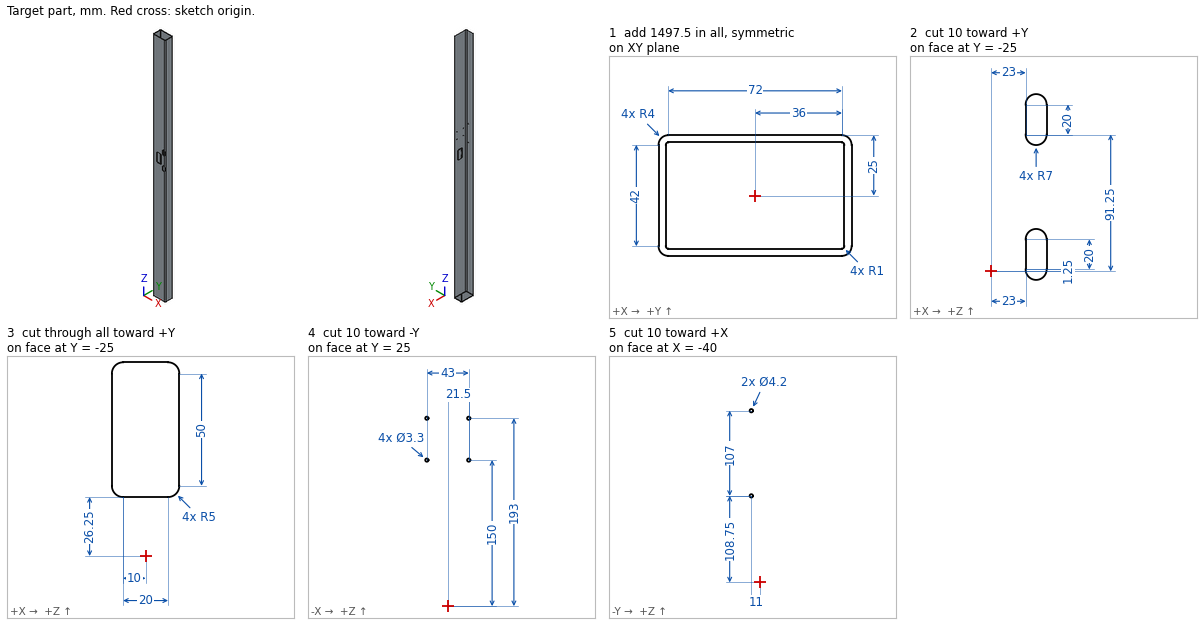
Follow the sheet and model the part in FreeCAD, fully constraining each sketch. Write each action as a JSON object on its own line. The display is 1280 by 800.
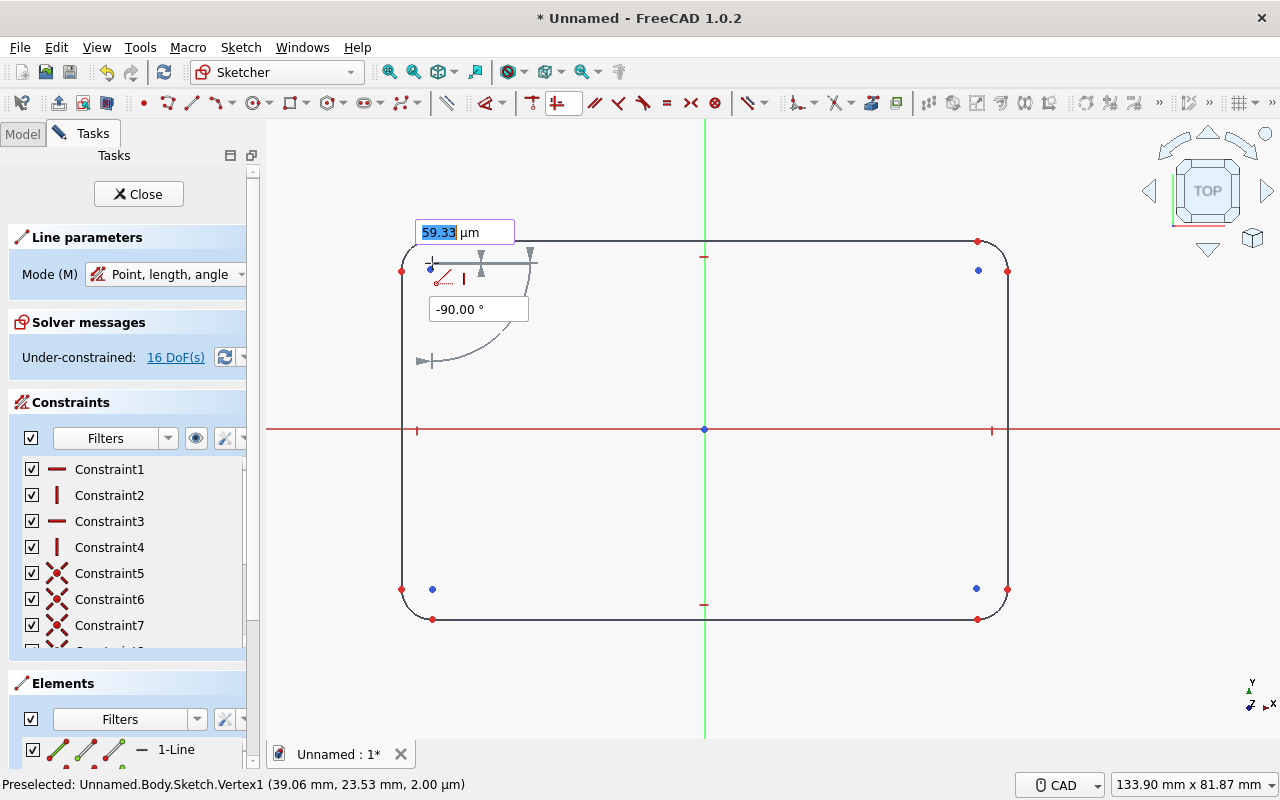
{"action": "scroll", "coordinate": [977, 263], "scroll_direction": "up", "scroll_amount": 4}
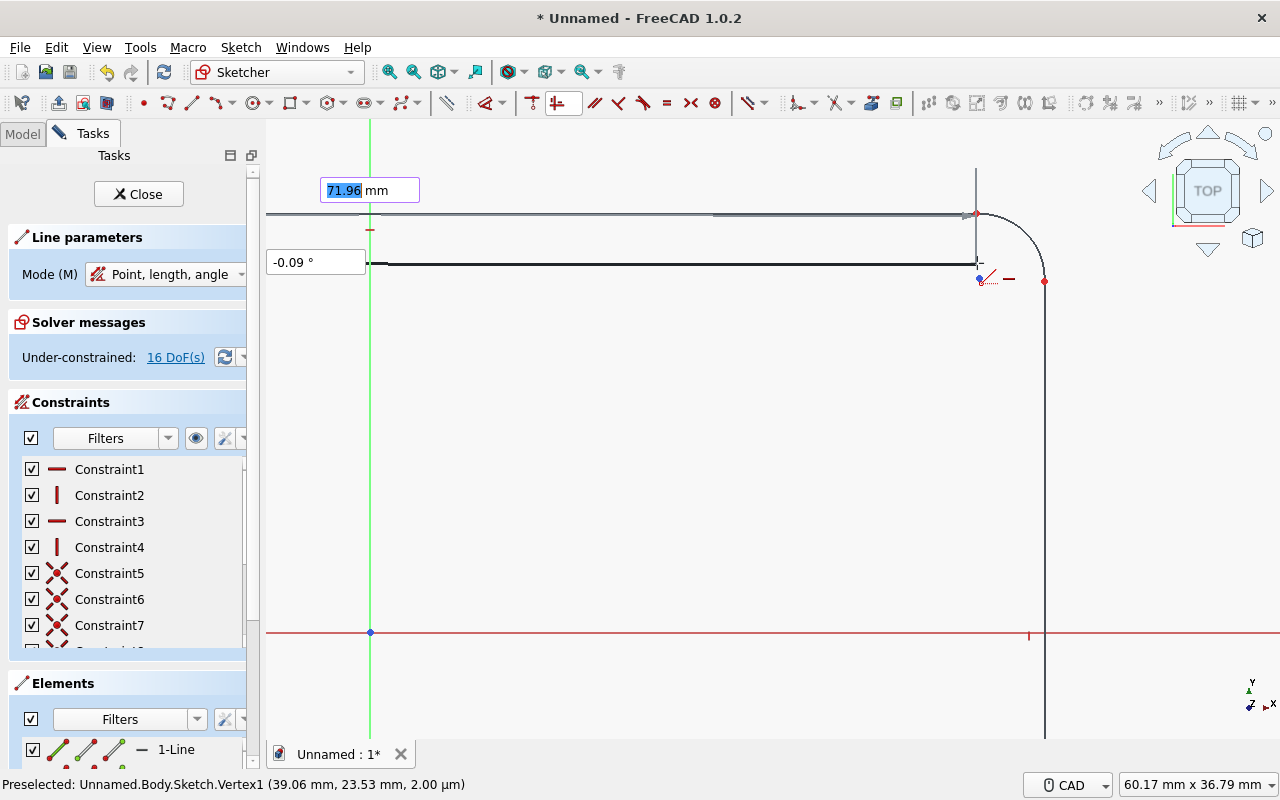
{"action": "left_click", "coordinate": [977, 262]}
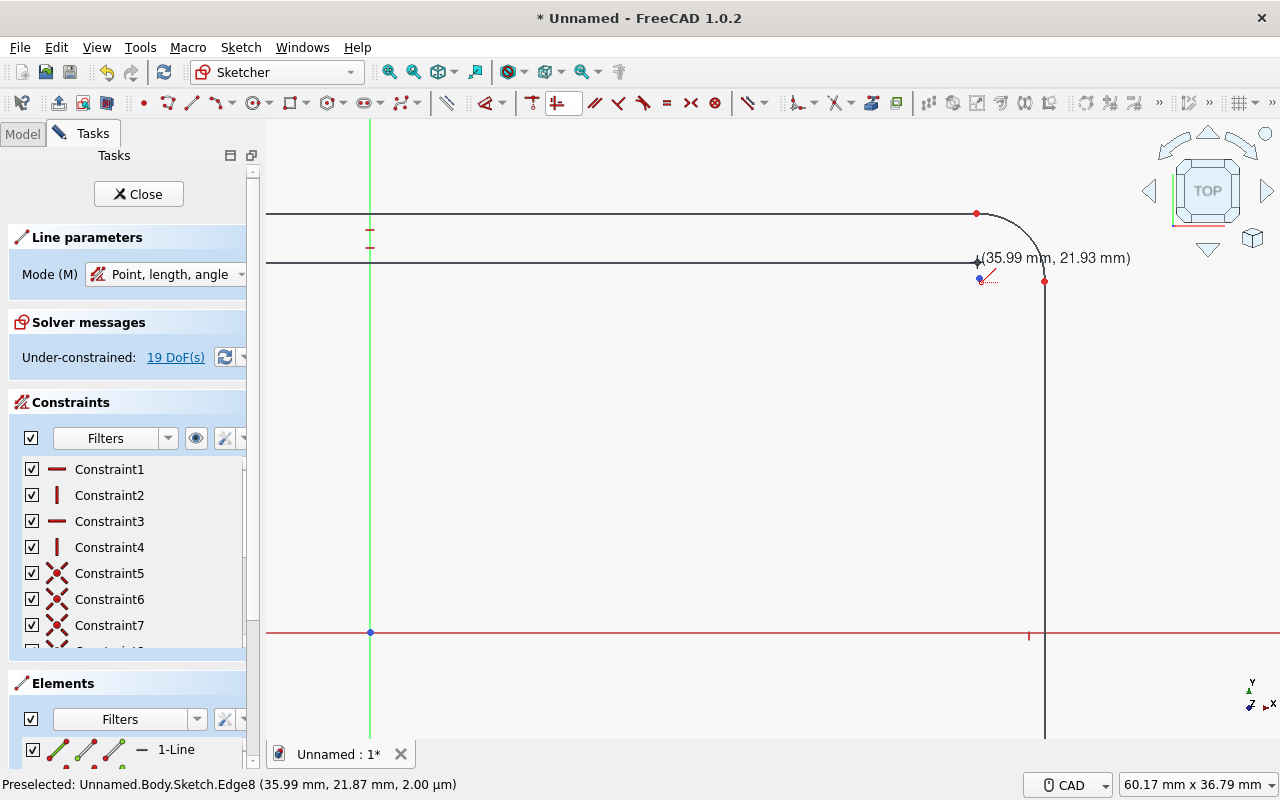
{"action": "left_click", "coordinate": [994, 279]}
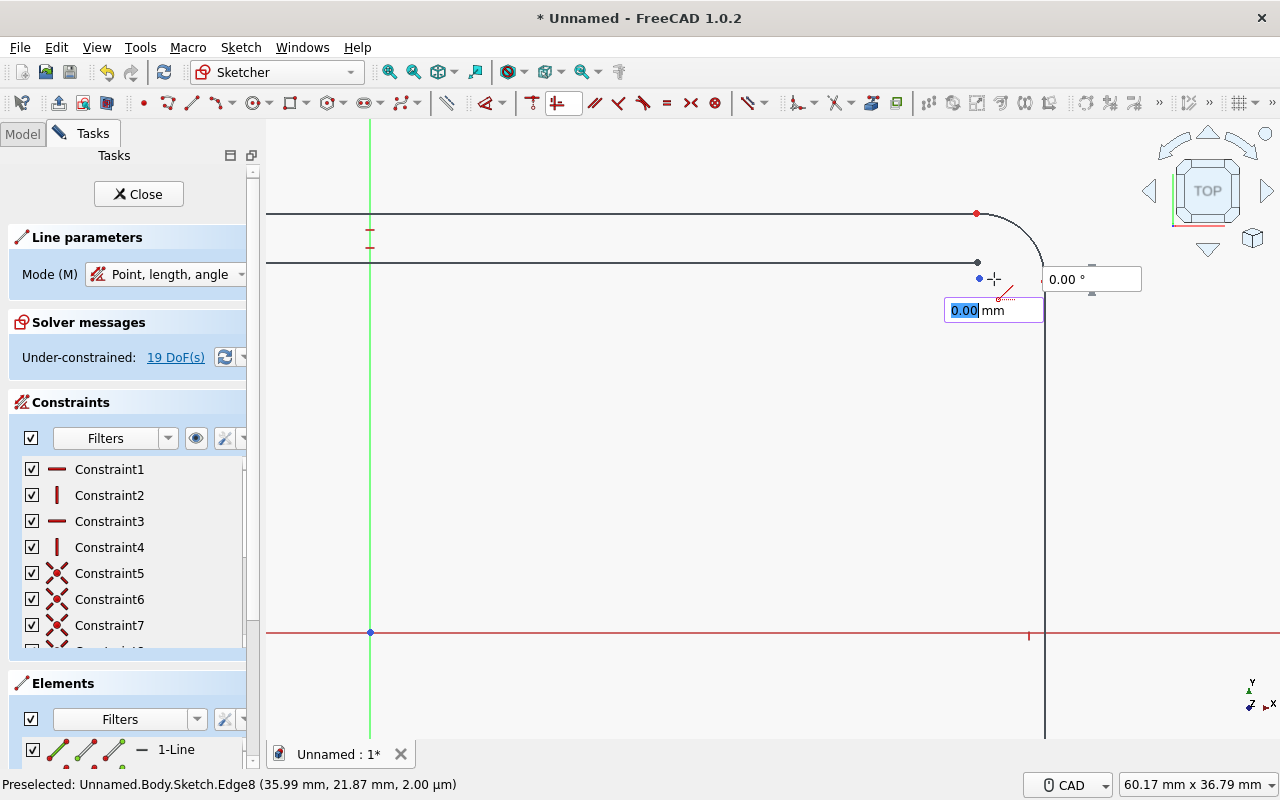
{"action": "scroll", "coordinate": [977, 263], "scroll_direction": "down", "scroll_amount": 4}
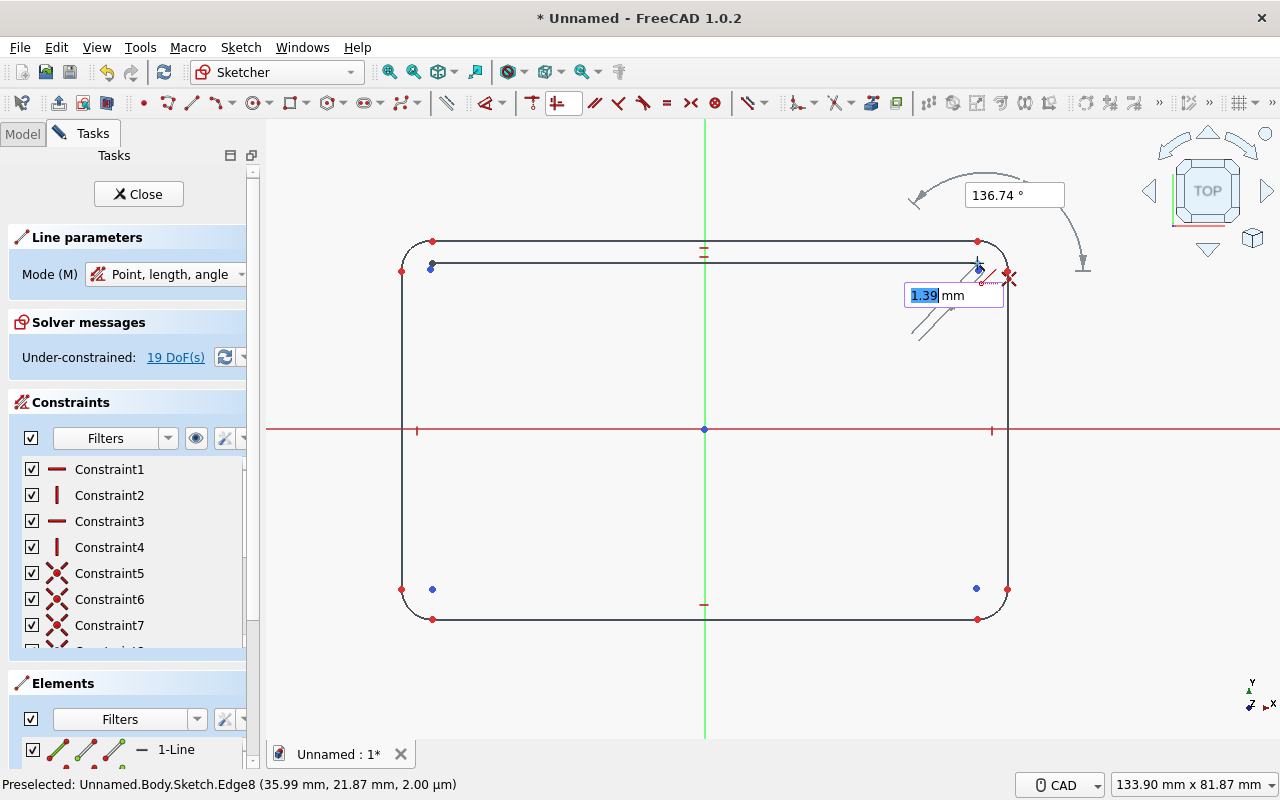
{"action": "scroll", "coordinate": [985, 588], "scroll_direction": "up", "scroll_amount": 4}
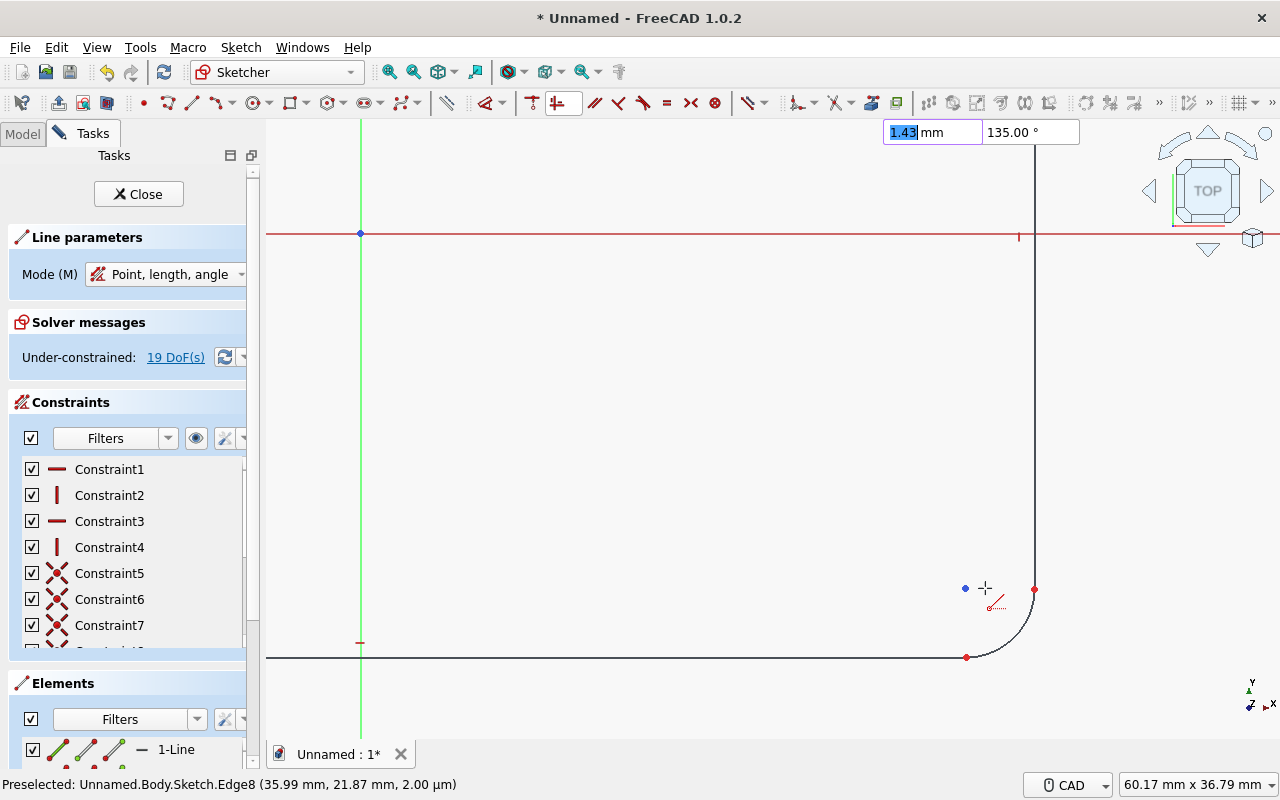
{"action": "left_click", "coordinate": [984, 588]}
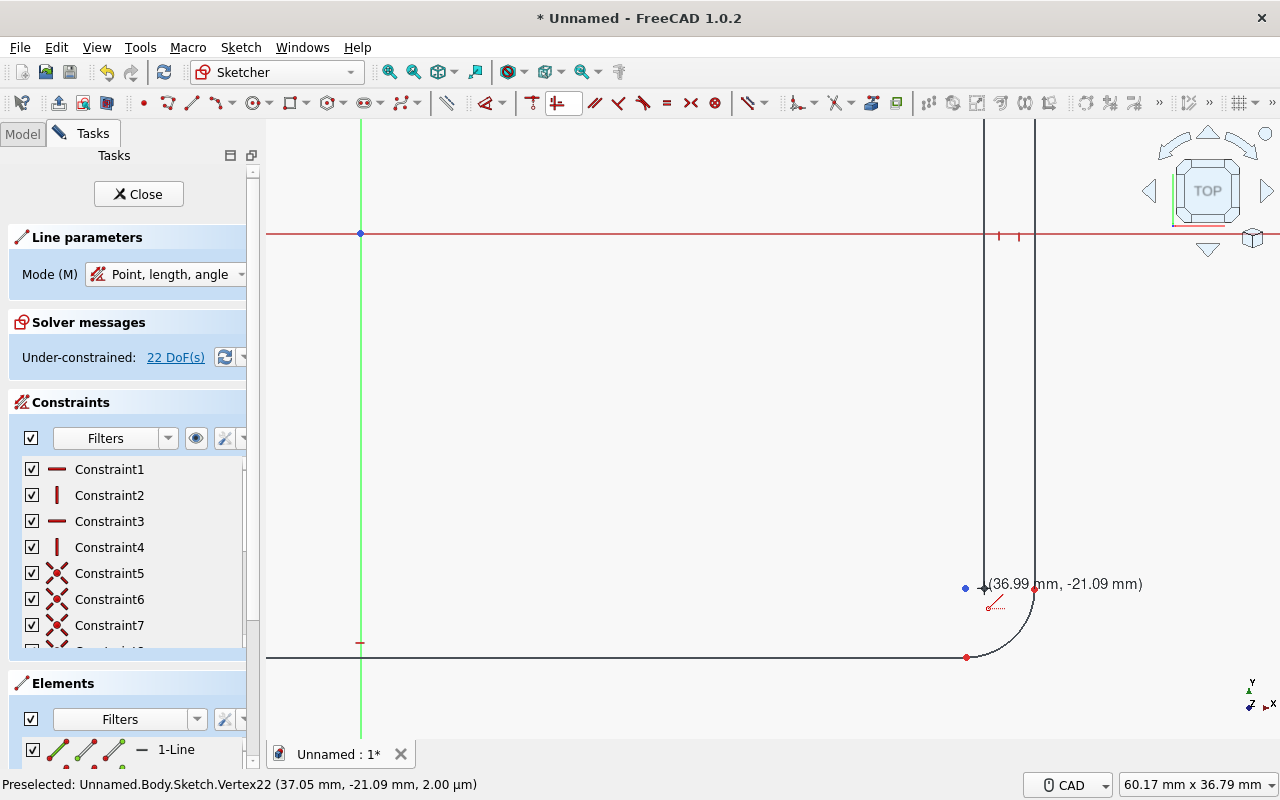
{"action": "left_click", "coordinate": [967, 604]}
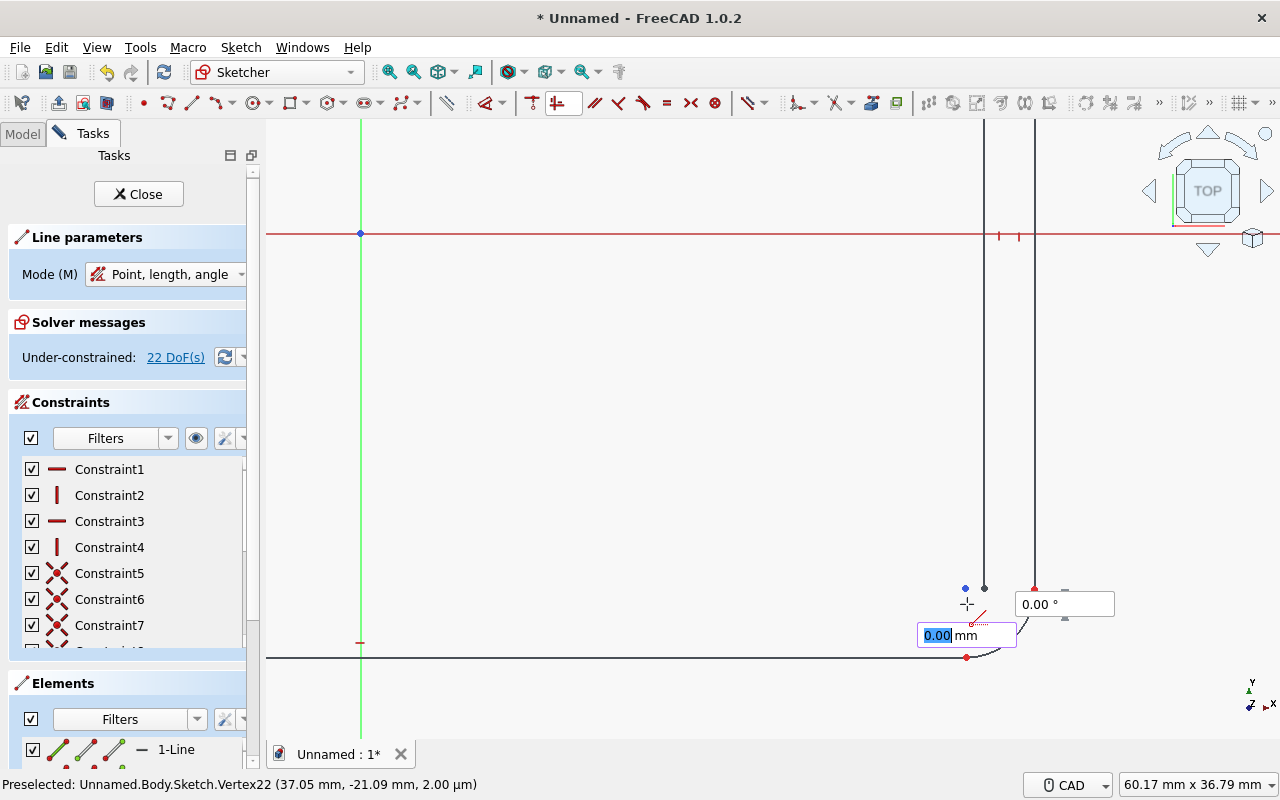
{"action": "scroll", "coordinate": [985, 588], "scroll_direction": "down", "scroll_amount": 4}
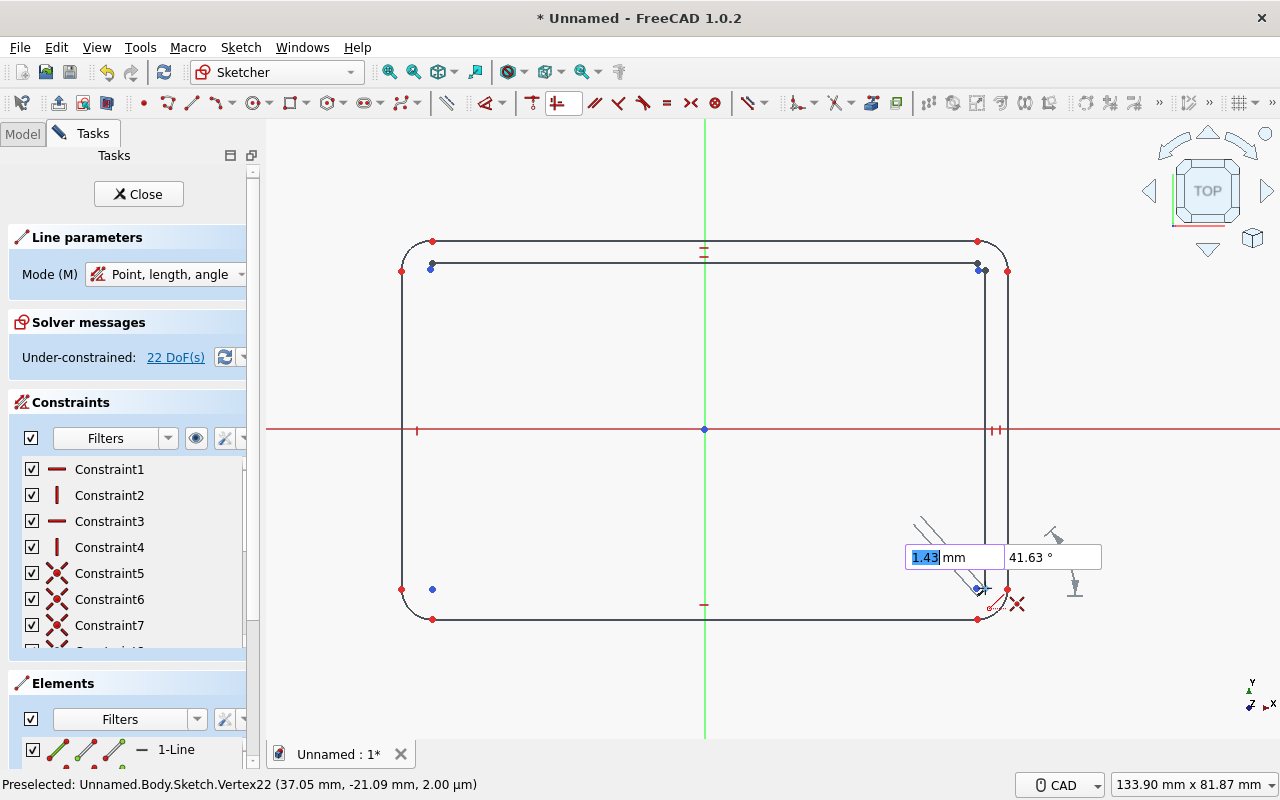
{"action": "scroll", "coordinate": [432, 596], "scroll_direction": "up", "scroll_amount": 4}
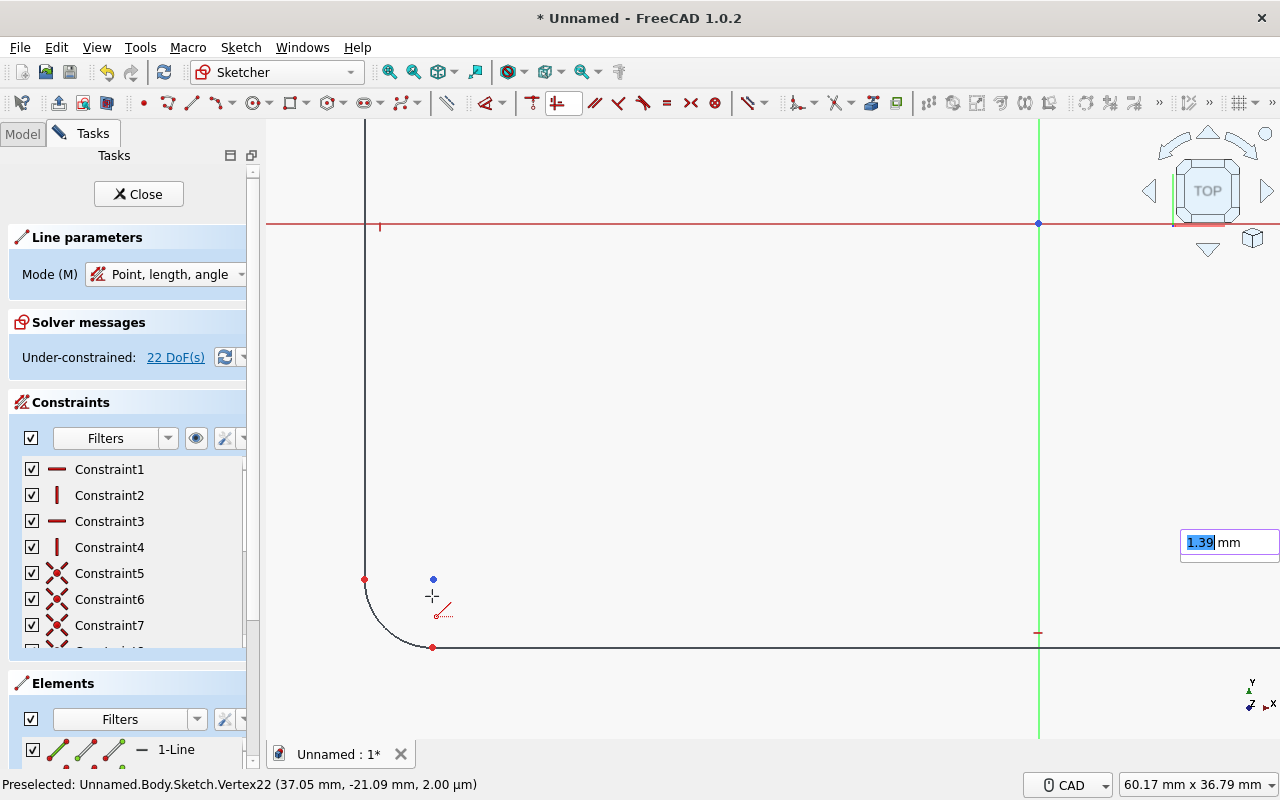
{"action": "left_click", "coordinate": [432, 594]}